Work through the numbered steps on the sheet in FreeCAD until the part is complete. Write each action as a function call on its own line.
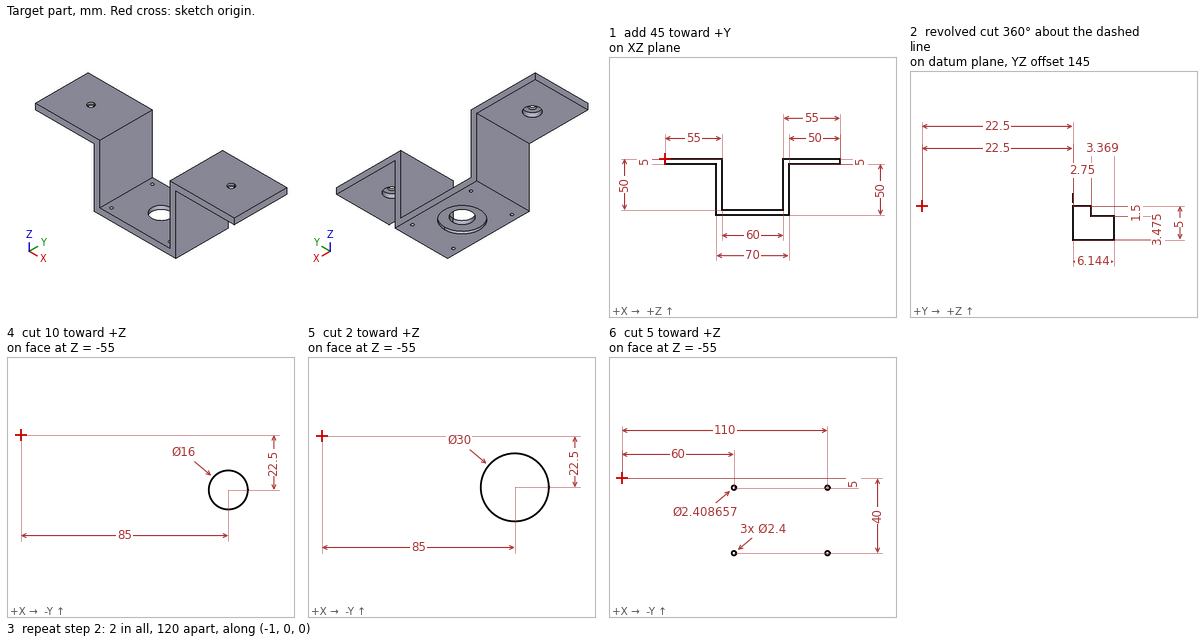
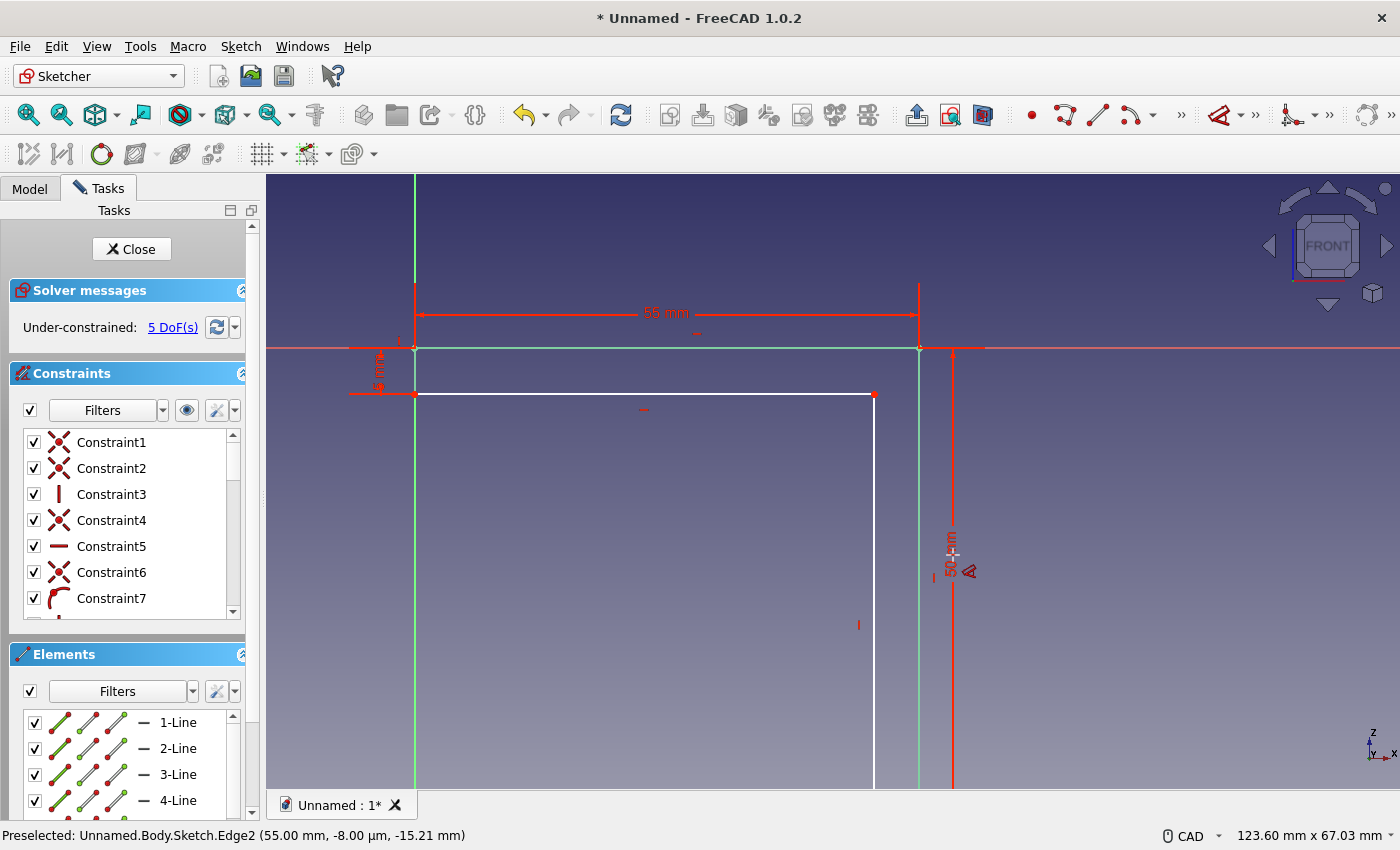
scroll(414, 384, down, 4)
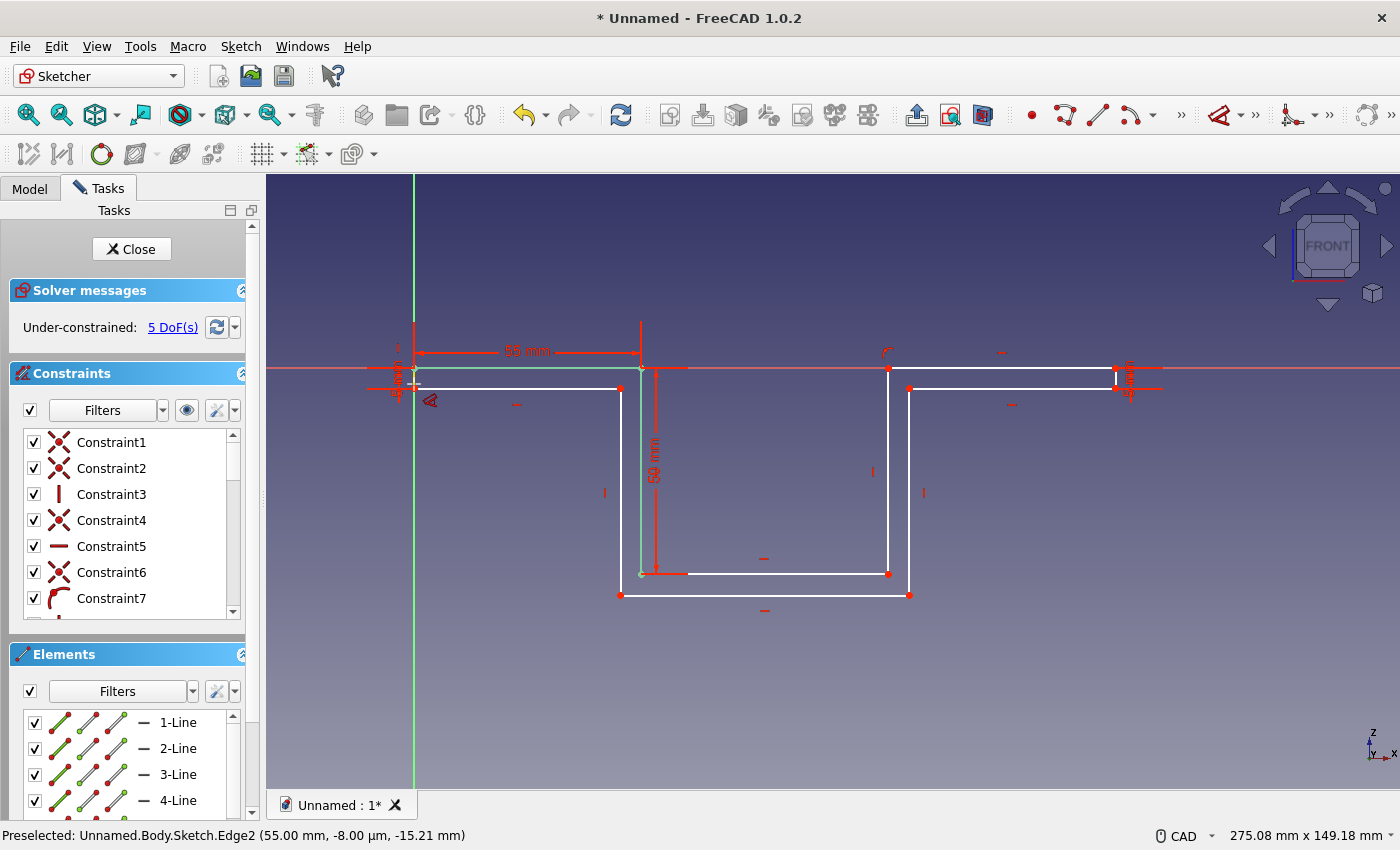
click(715, 574)
click(765, 540)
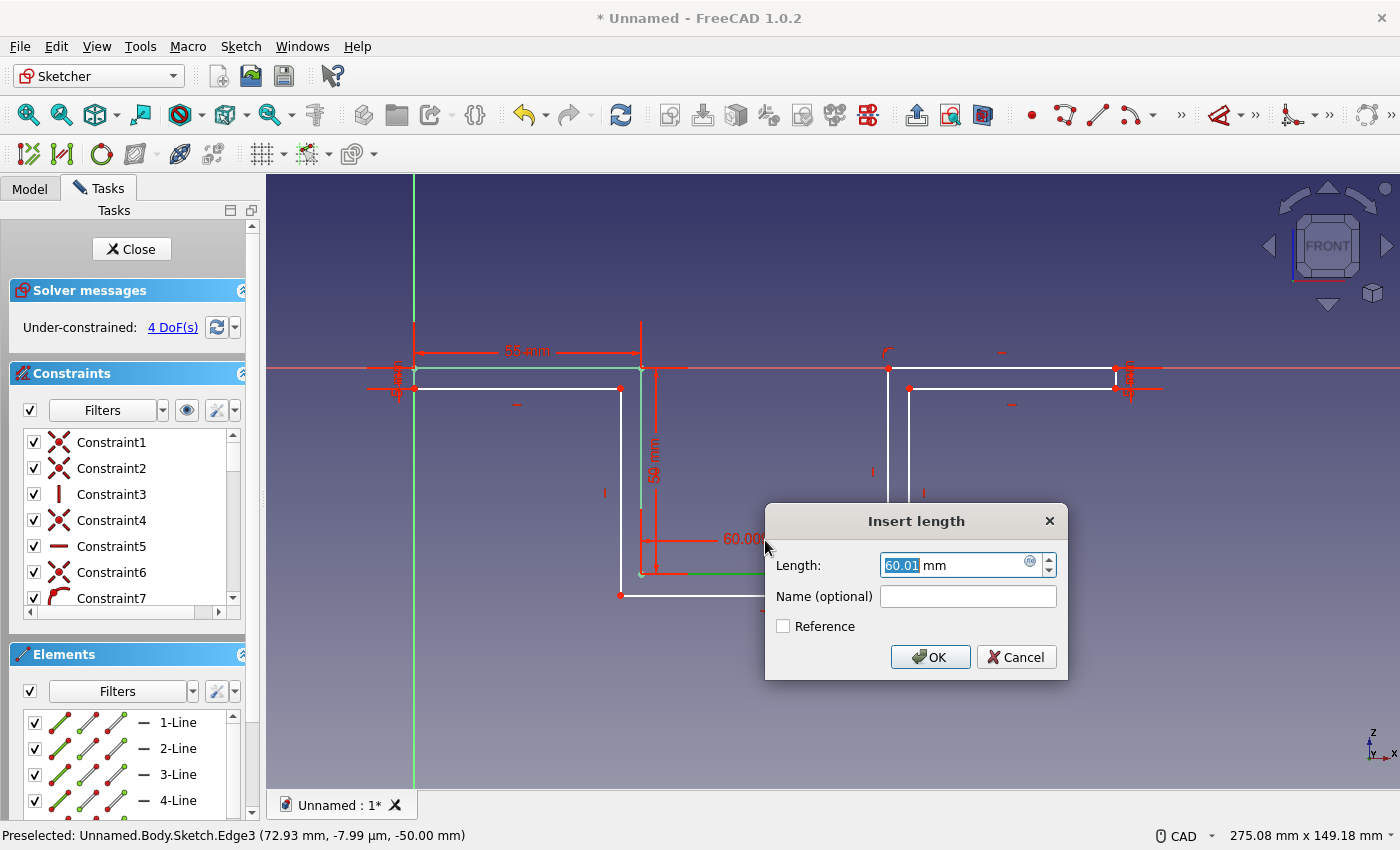
text(60)
key(Return)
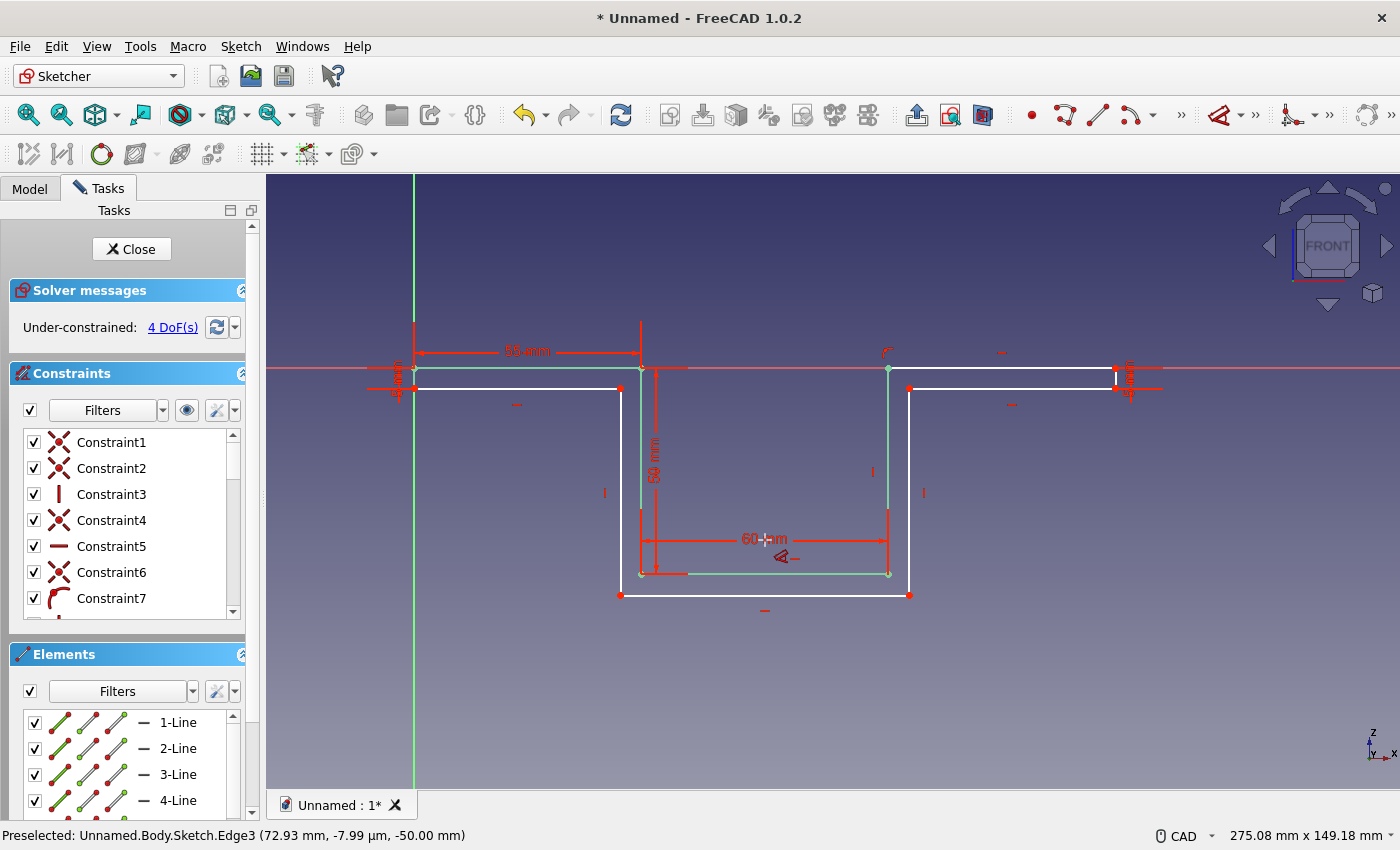
click(957, 368)
click(1002, 334)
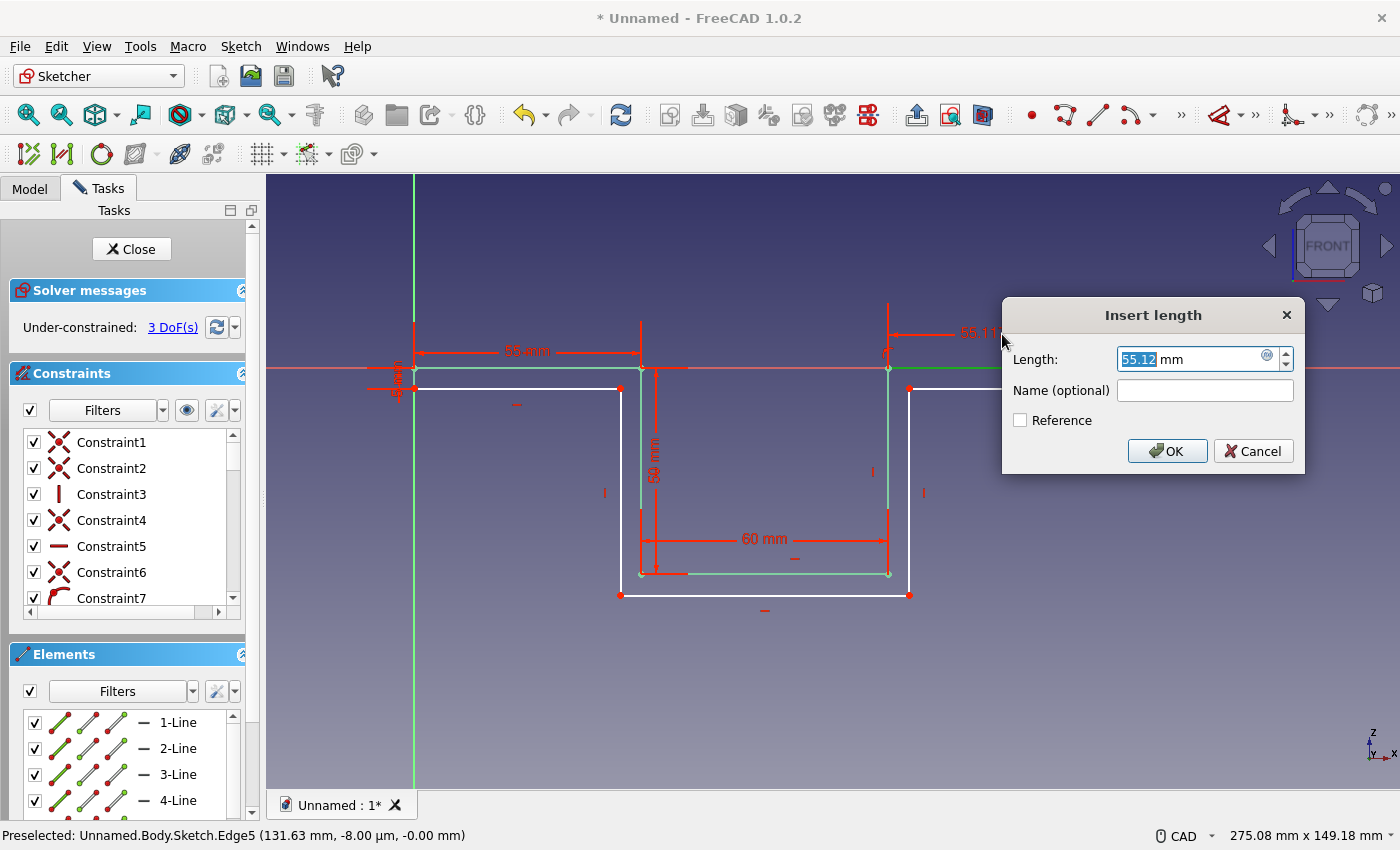
text(55)
key(Return)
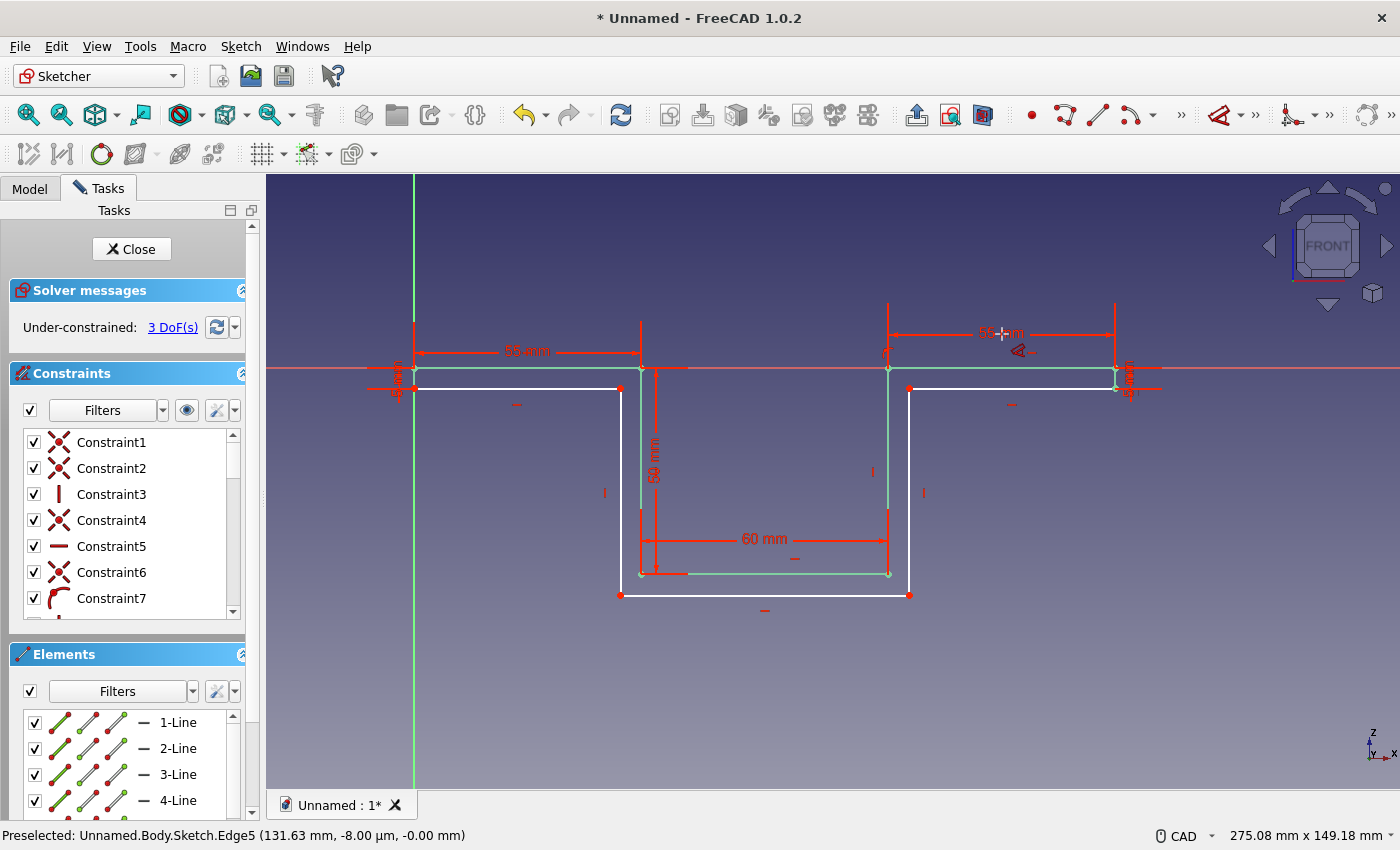
click(1053, 389)
click(1012, 355)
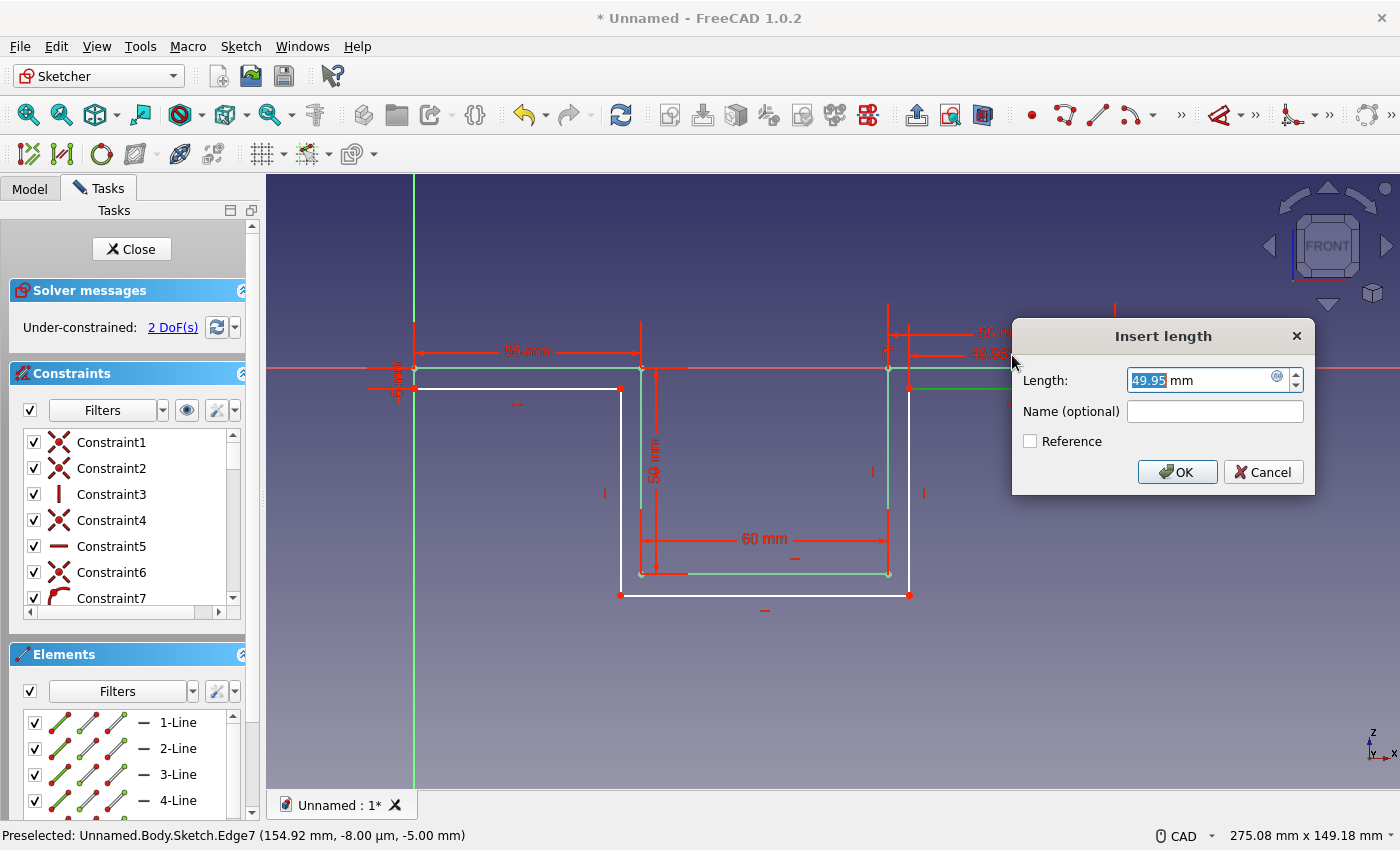
text(50)
key(Return)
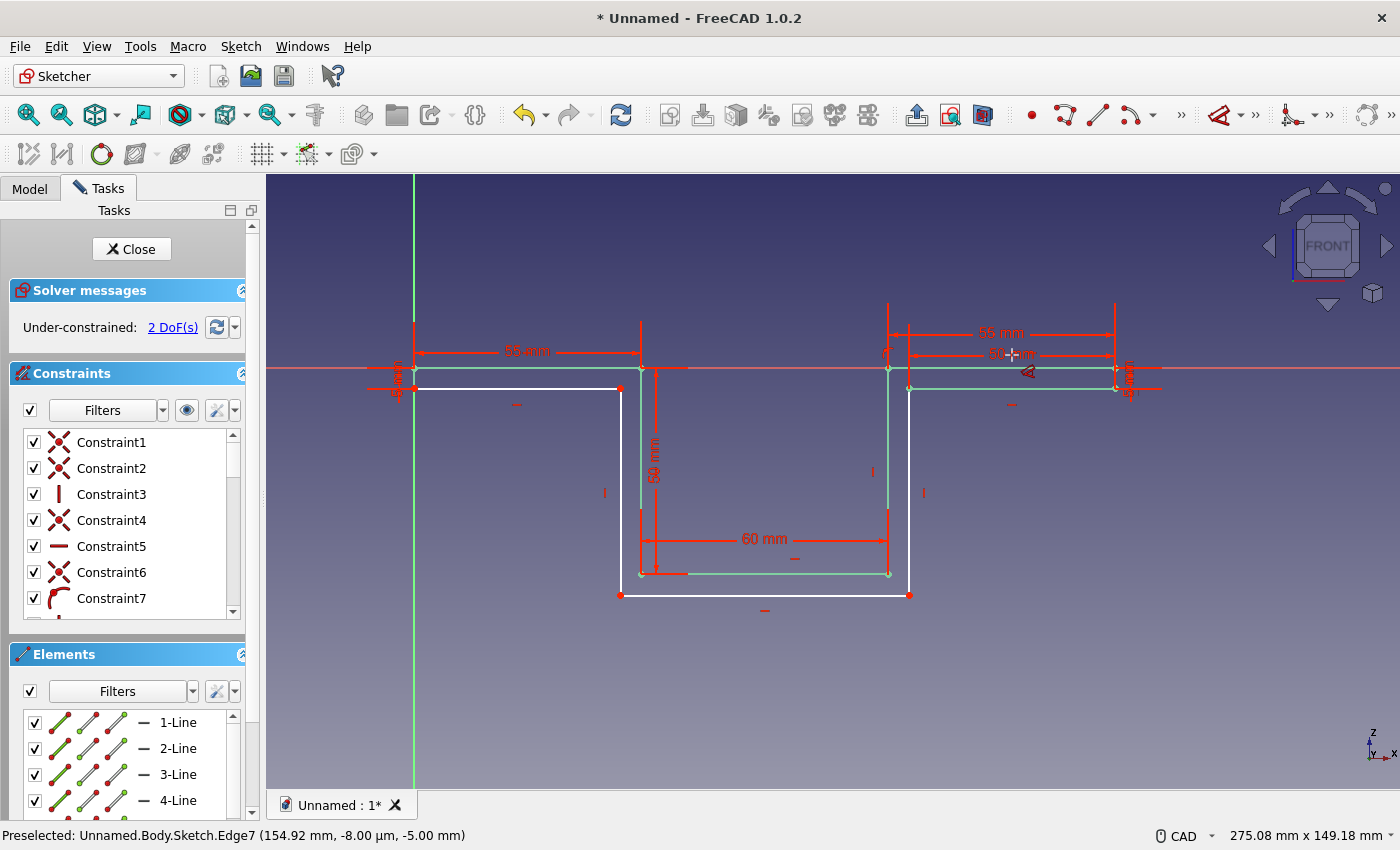
click(909, 451)
click(943, 492)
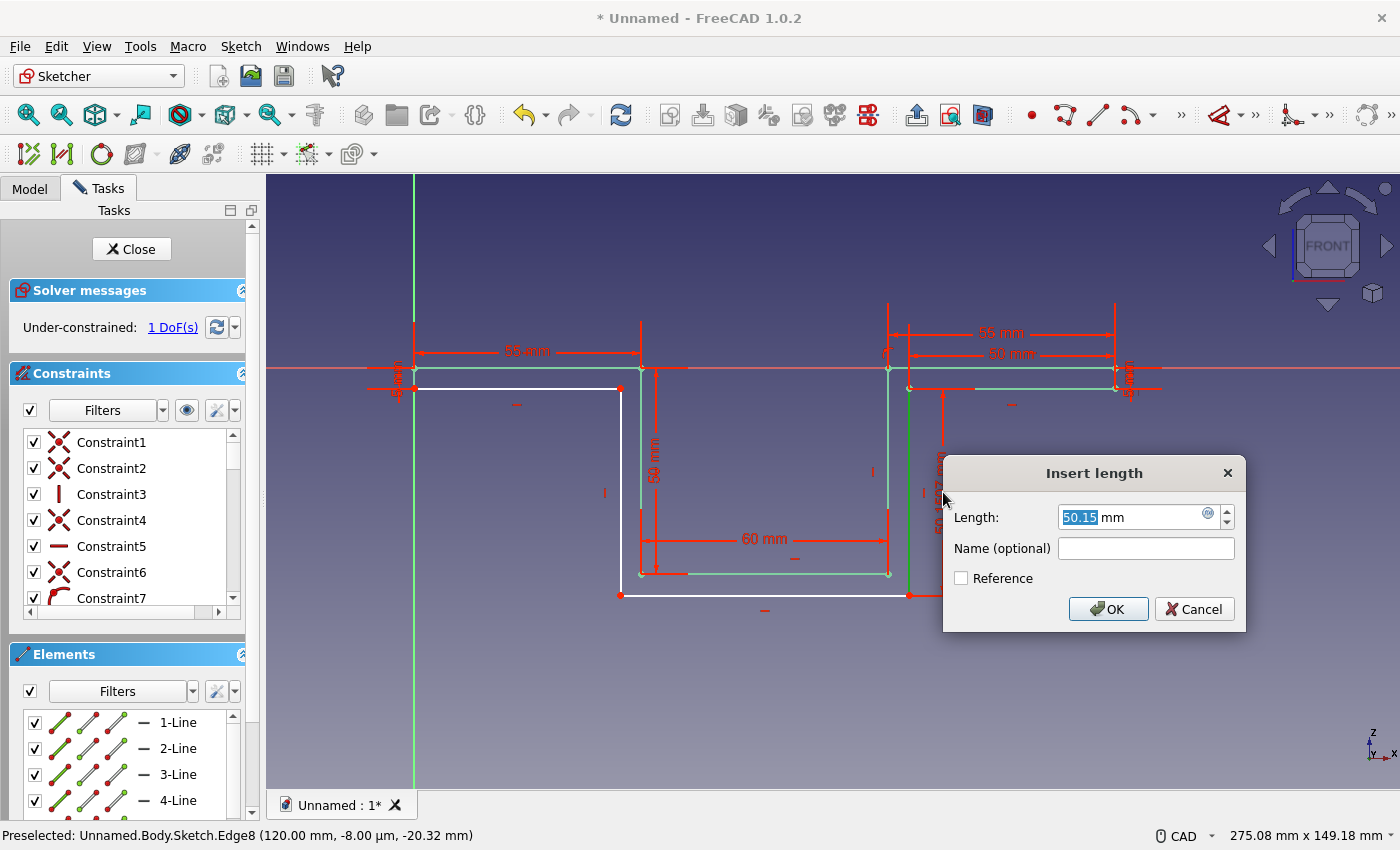
text(50)
key(Return)